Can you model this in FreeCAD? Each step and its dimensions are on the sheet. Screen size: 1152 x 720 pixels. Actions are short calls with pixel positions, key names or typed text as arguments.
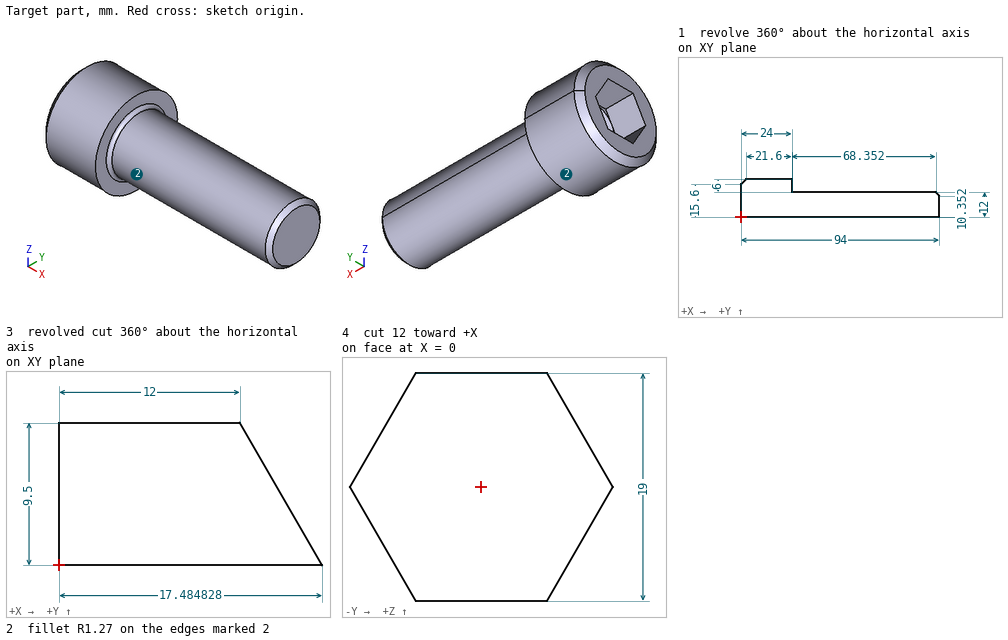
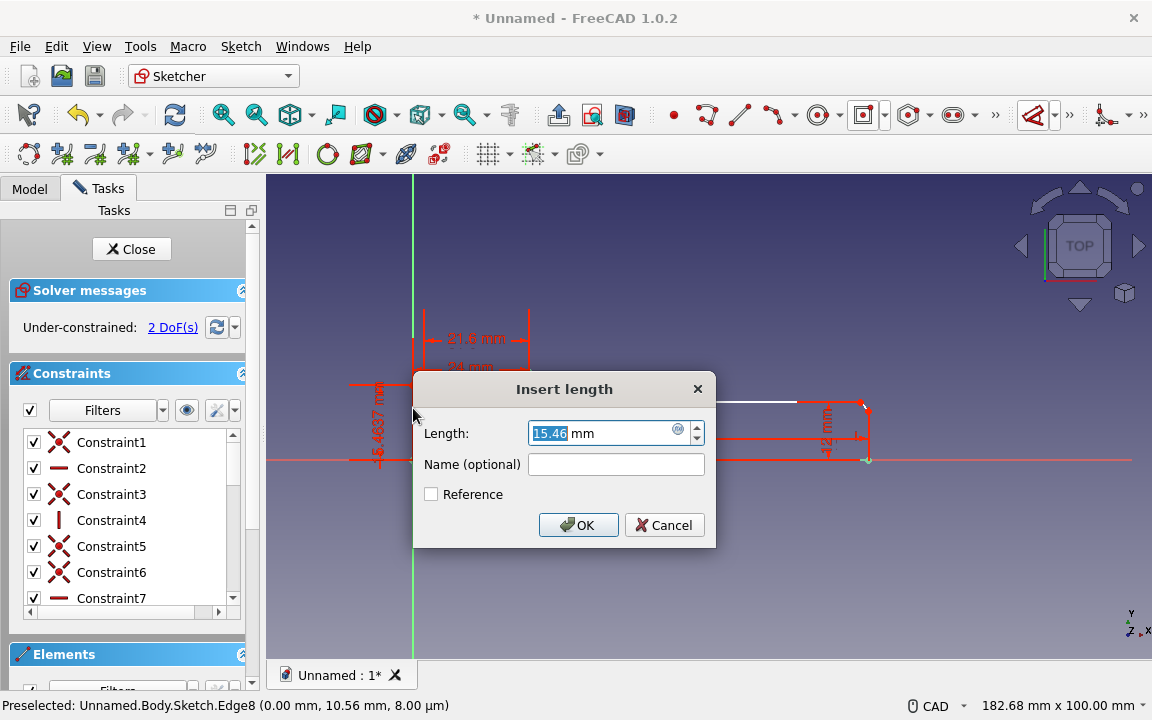
text(15.6)
key(Return)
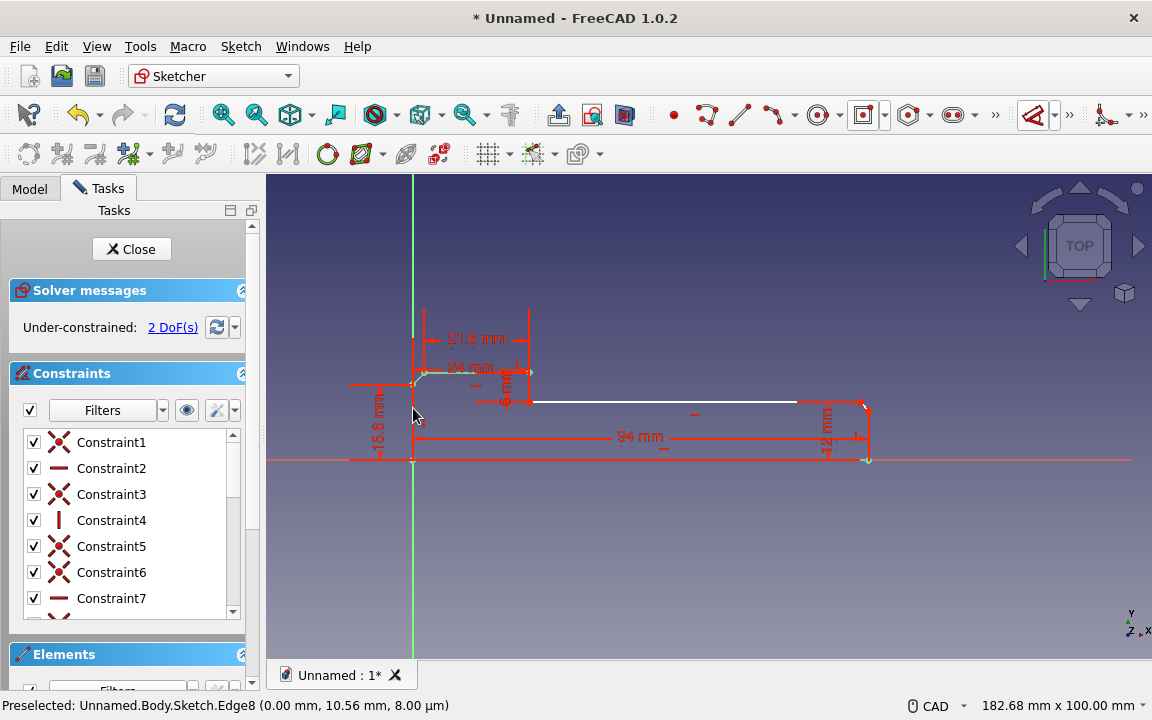
click(869, 446)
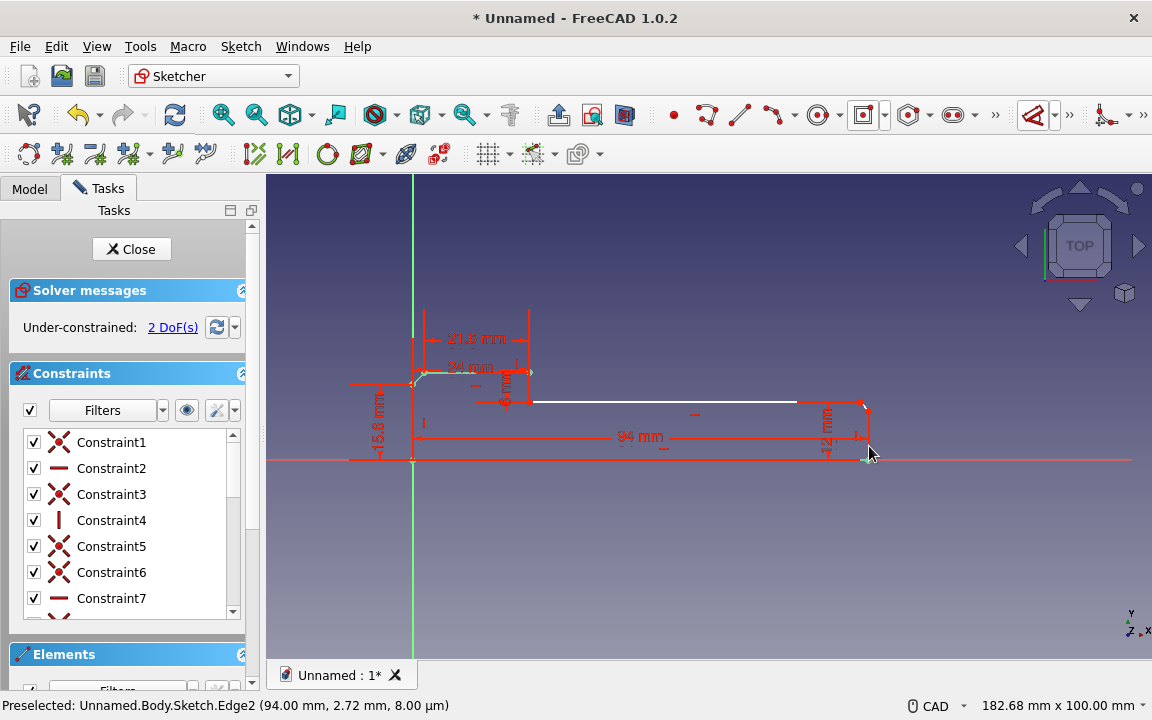
click(1054, 116)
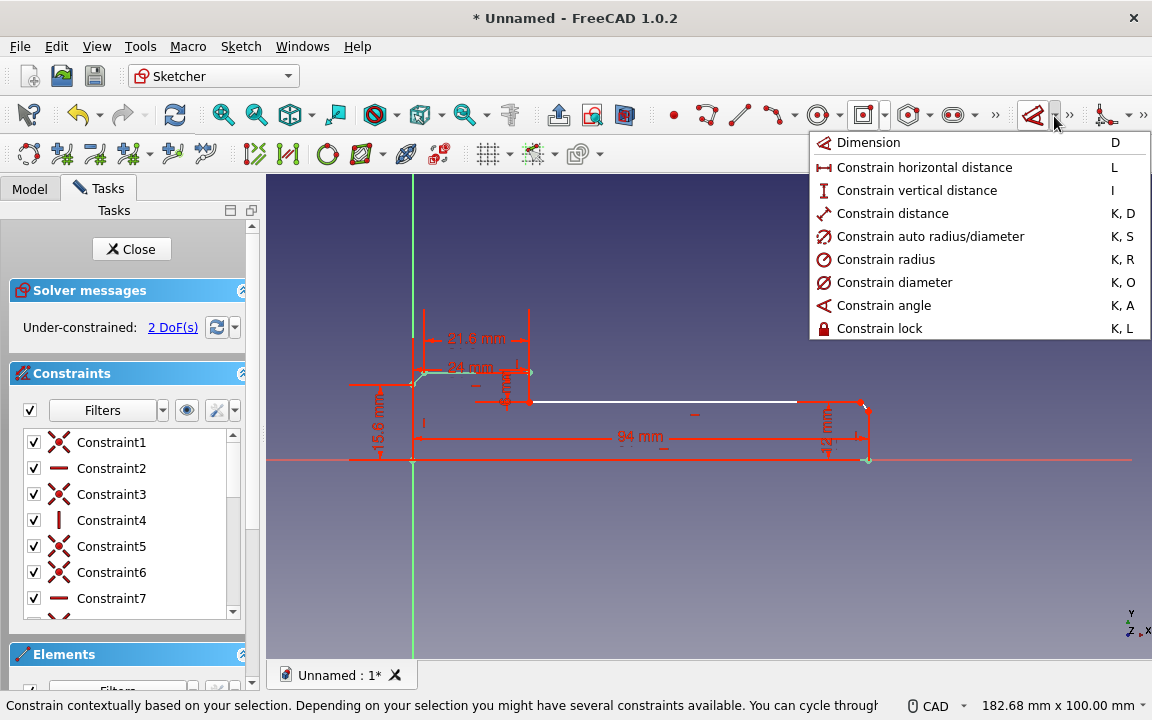
click(980, 190)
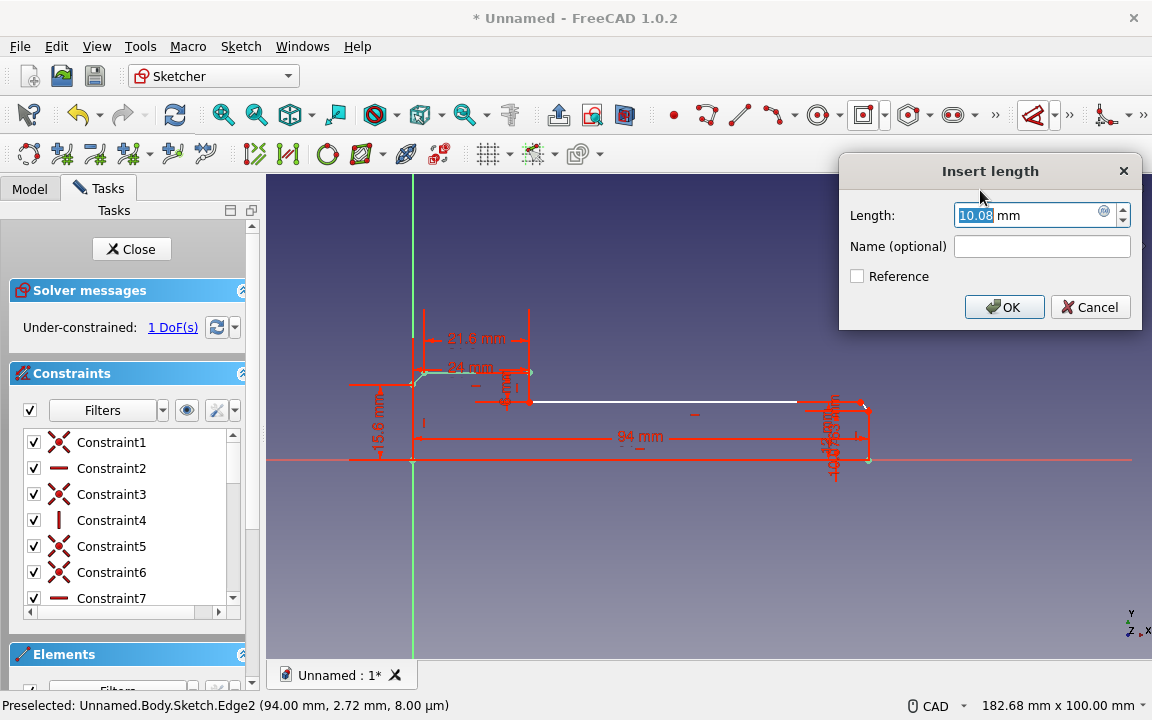
text(10.352)
key(Return)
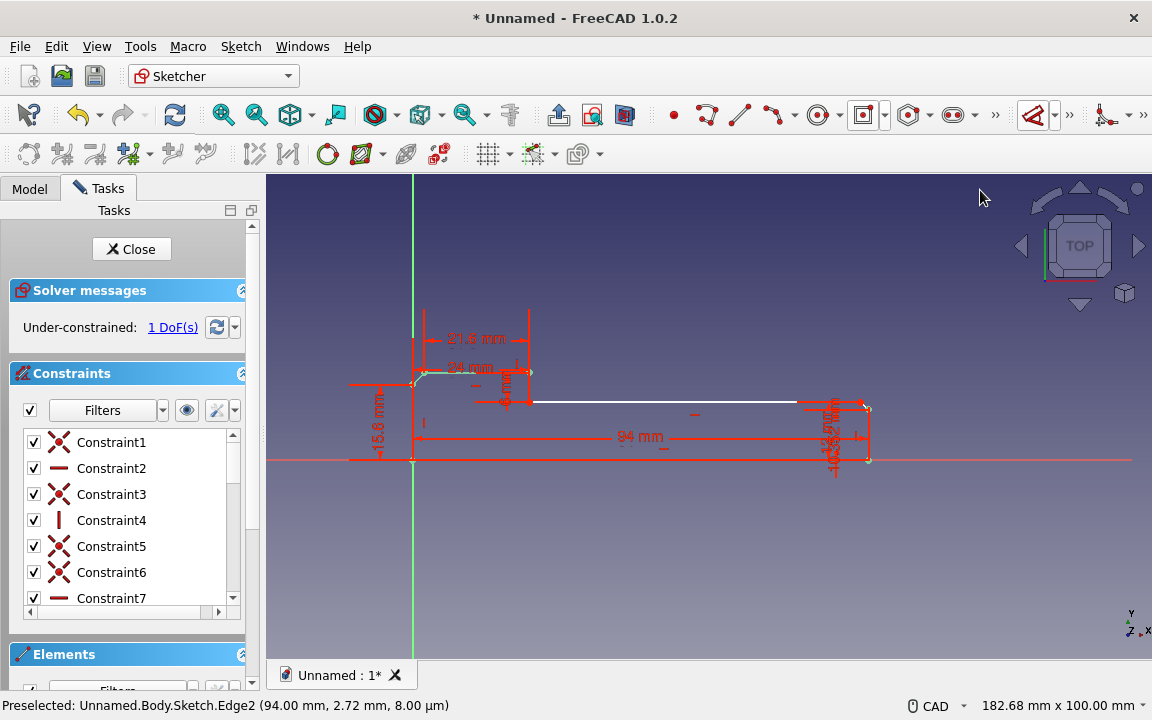
click(761, 402)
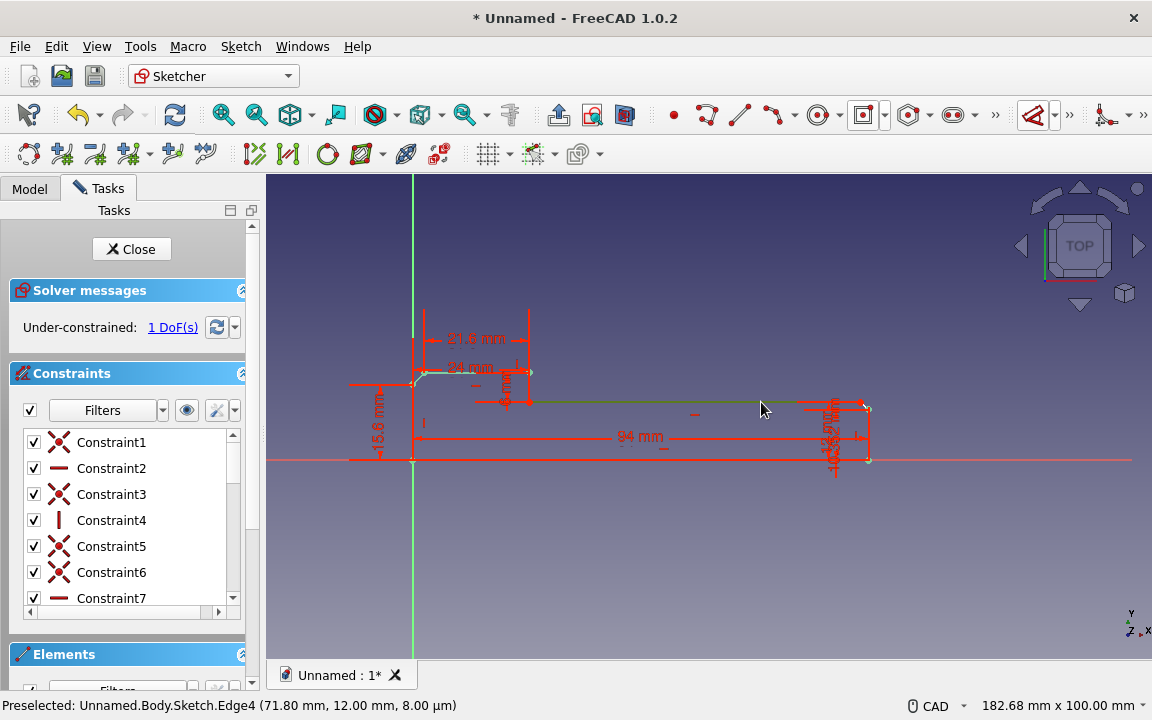
click(1054, 116)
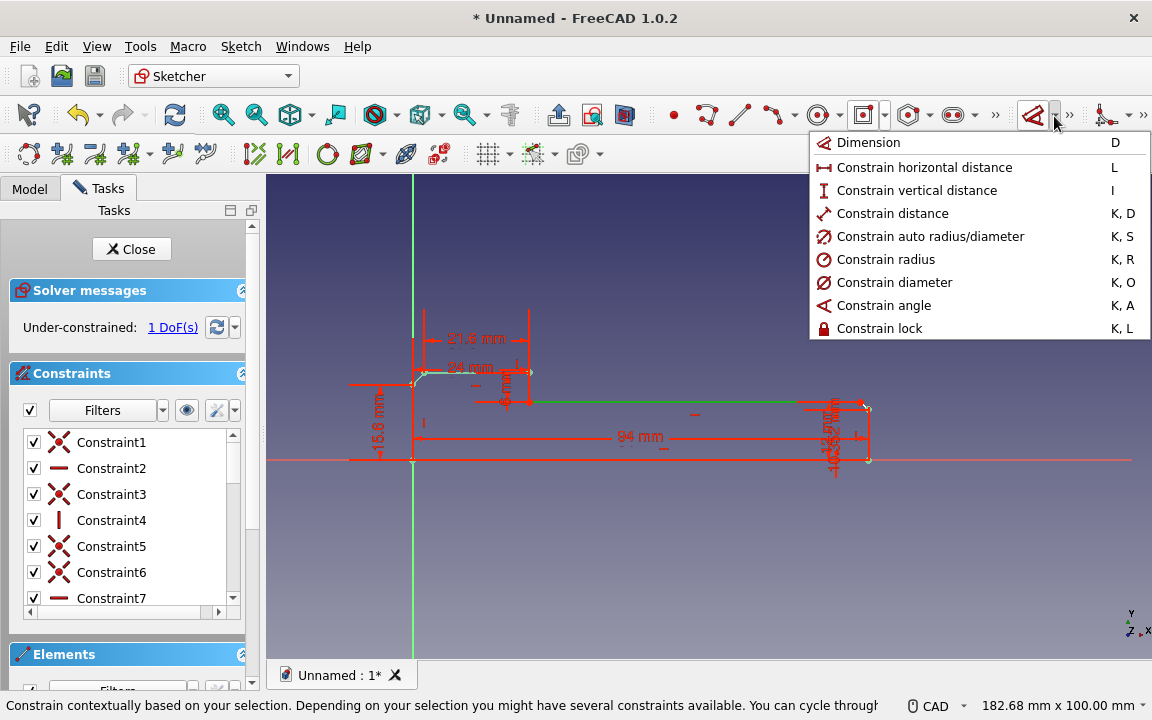
click(980, 168)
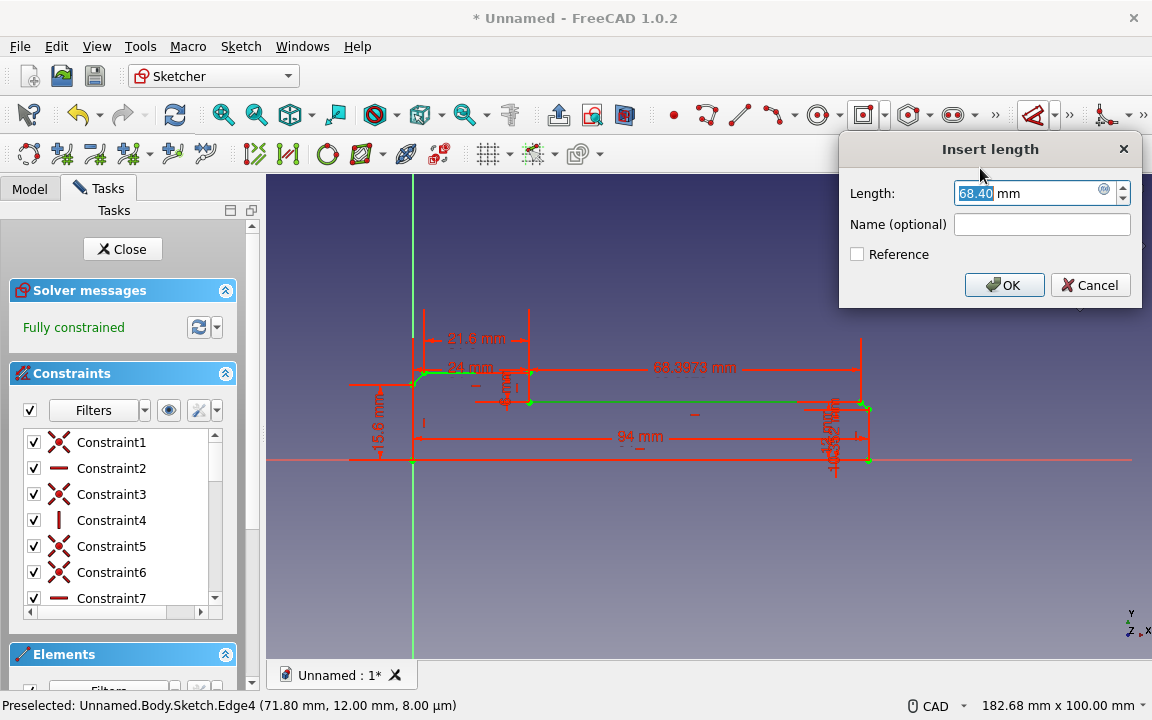
text(68.352)
key(Return)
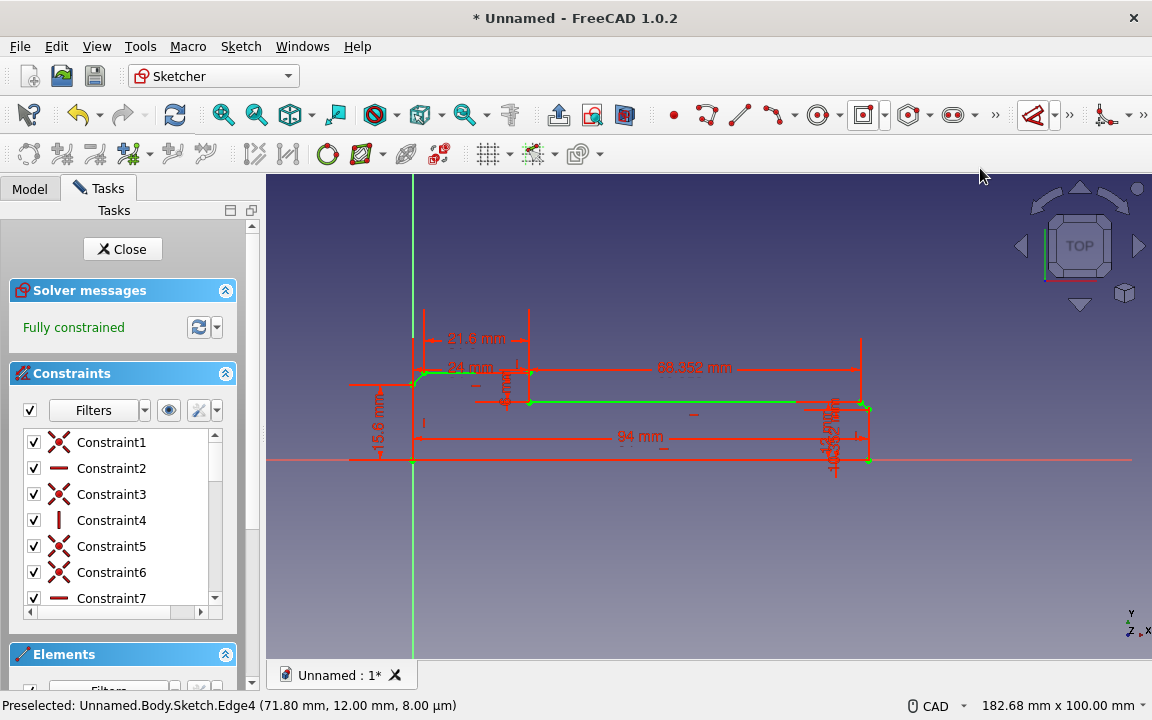
click(123, 249)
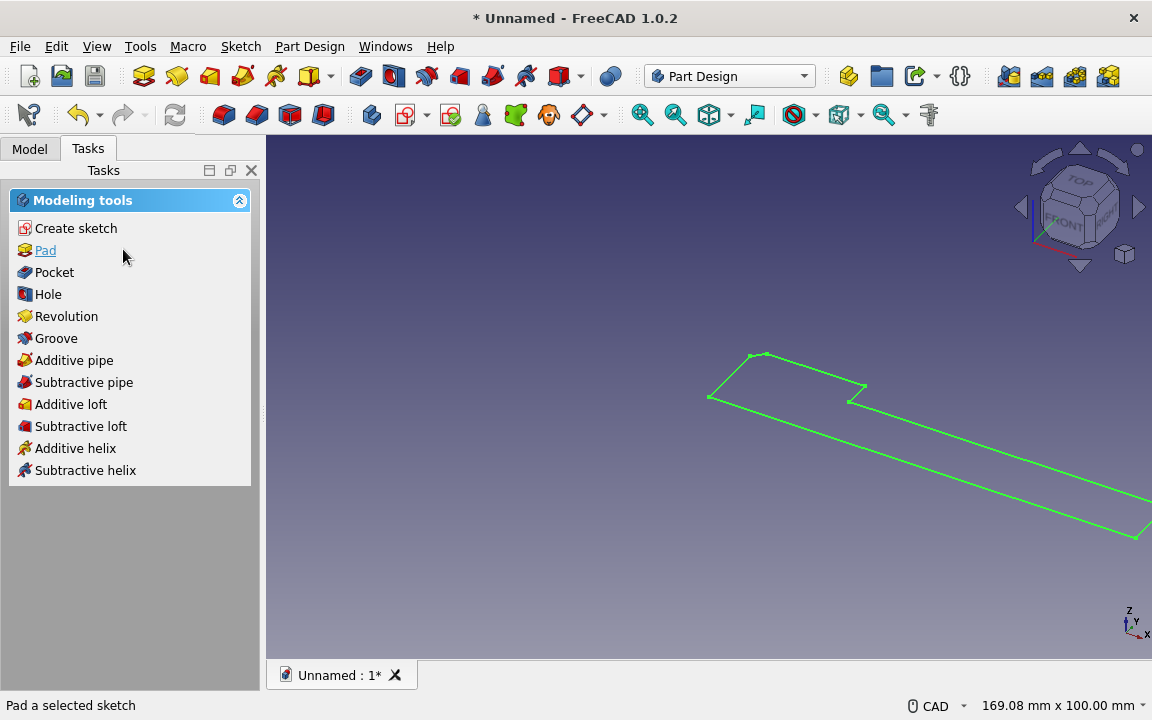
click(177, 76)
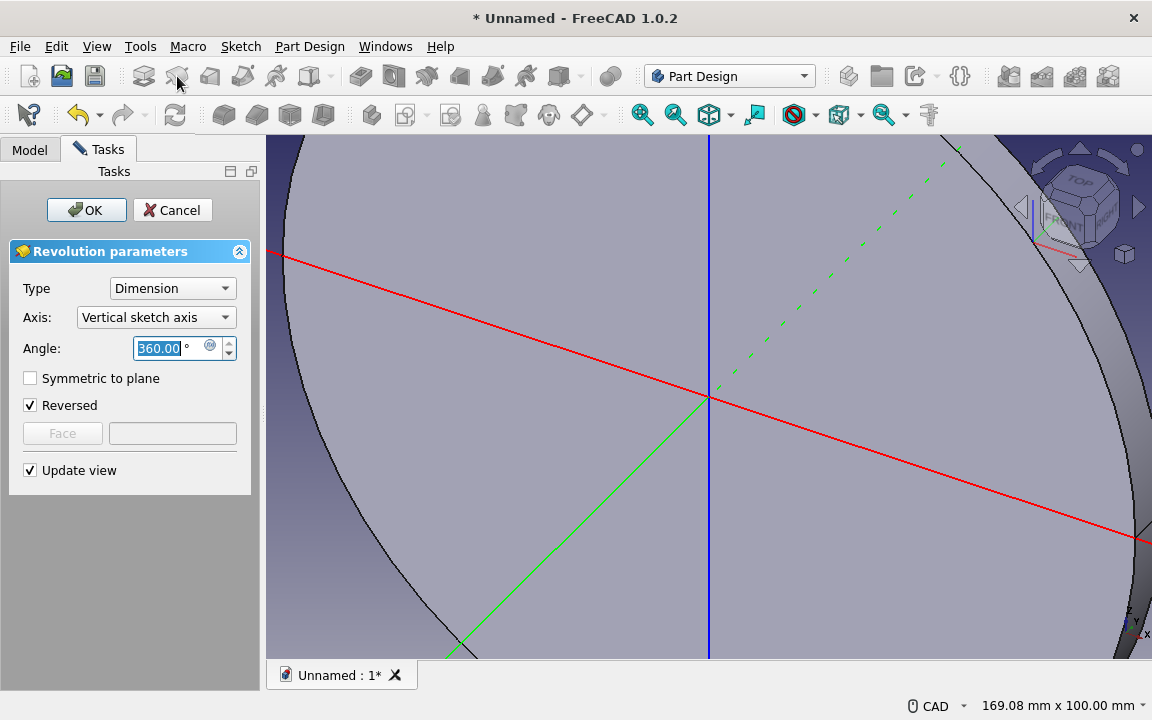
click(157, 318)